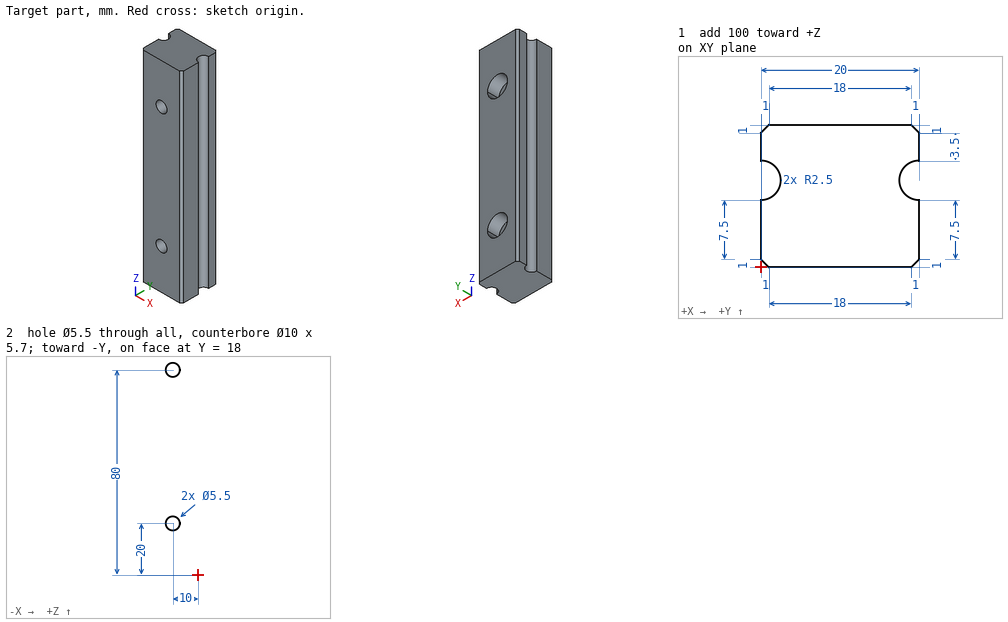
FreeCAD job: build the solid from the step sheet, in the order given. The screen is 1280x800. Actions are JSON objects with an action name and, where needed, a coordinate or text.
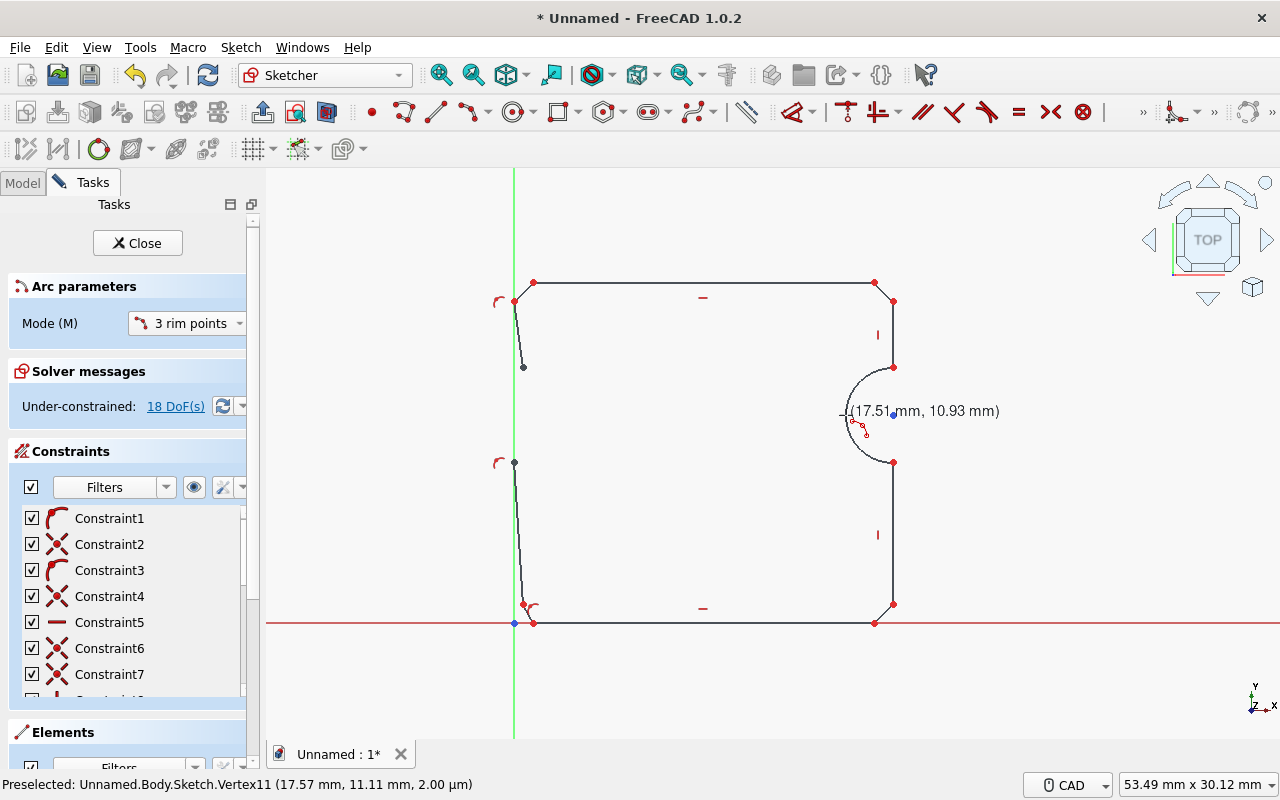
{"action": "left_click", "coordinate": [523, 368]}
{"action": "left_click", "coordinate": [514, 463]}
{"action": "left_click", "coordinate": [561, 415]}
{"action": "key", "text": "Escape"}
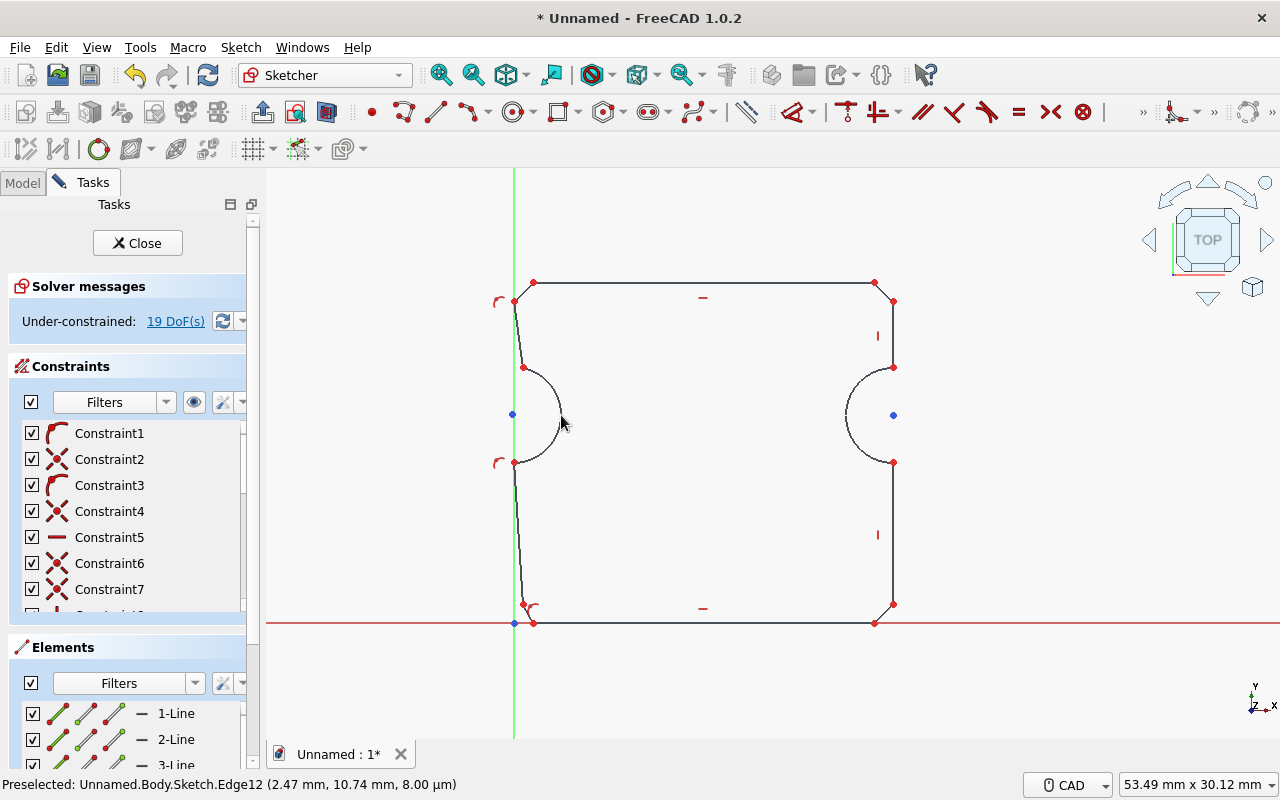
{"action": "left_click", "coordinate": [517, 506]}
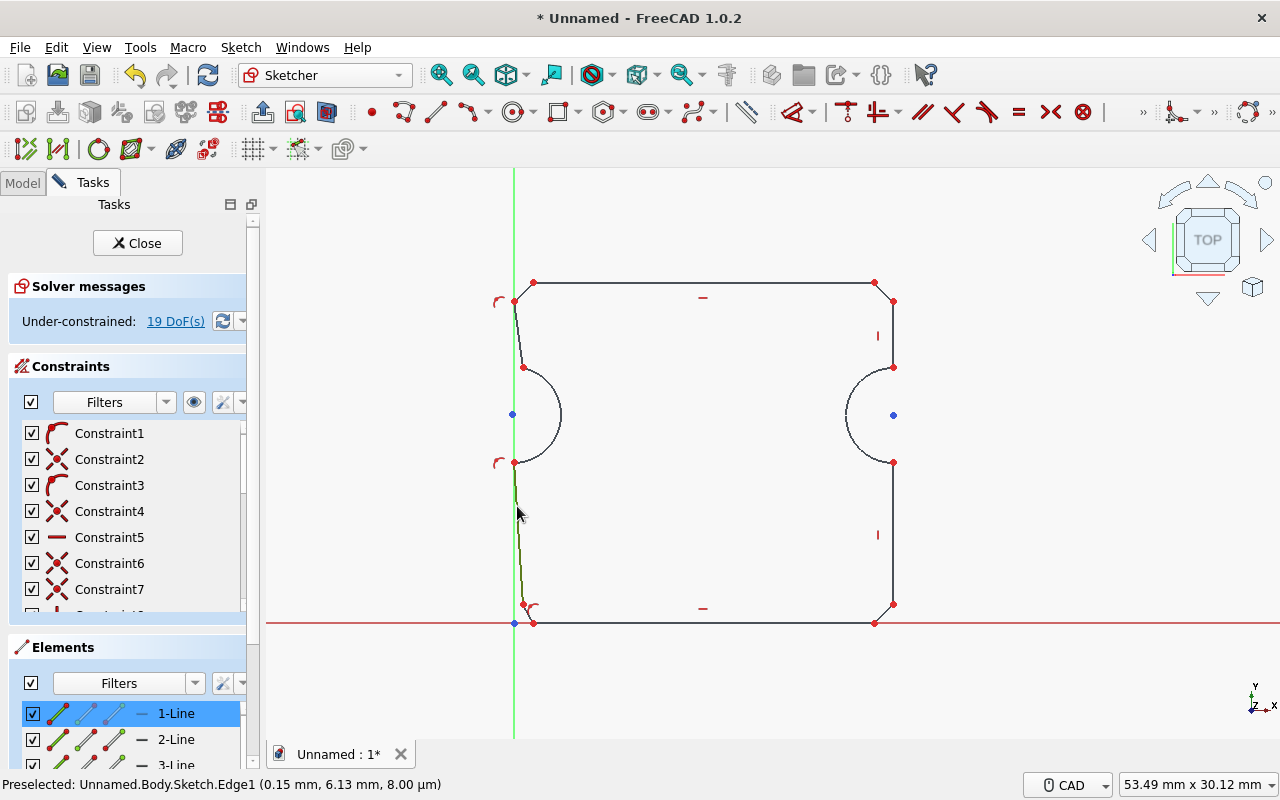
{"action": "key", "text": "v"}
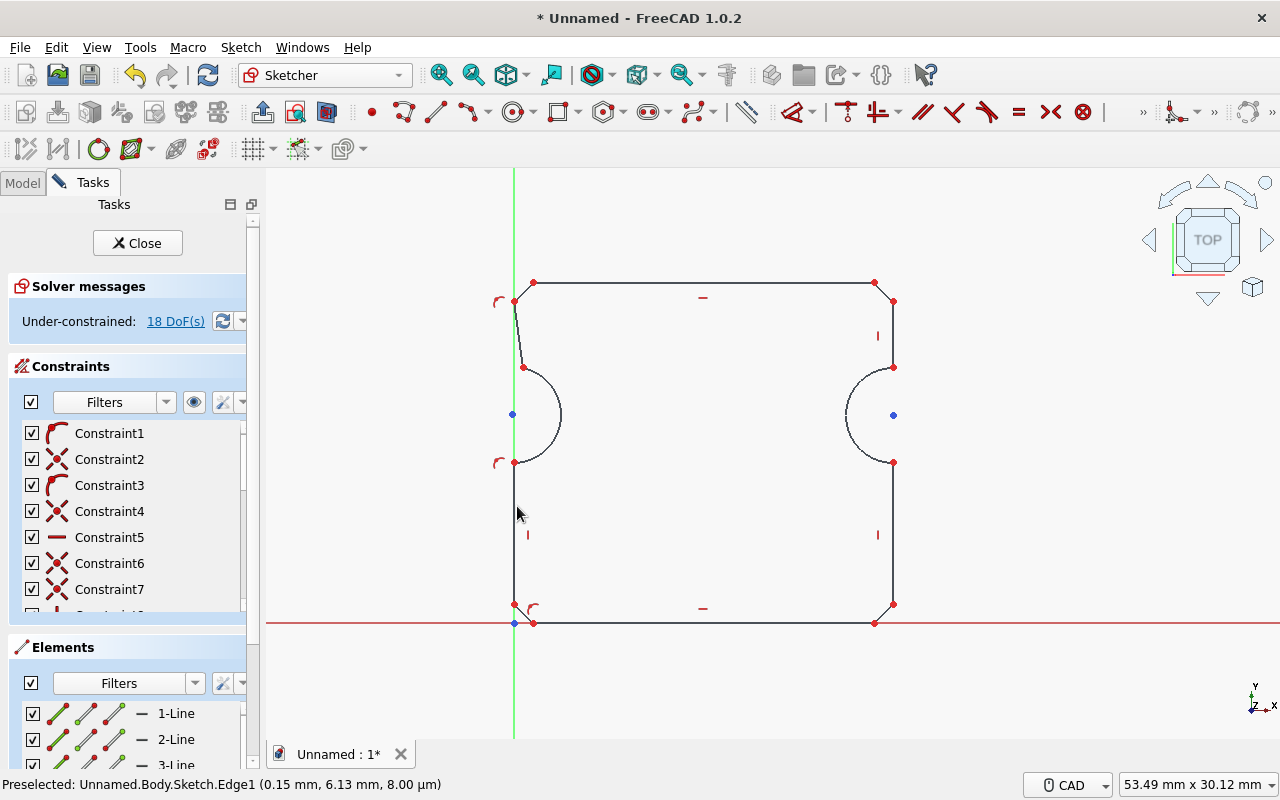
{"action": "left_click", "coordinate": [517, 322]}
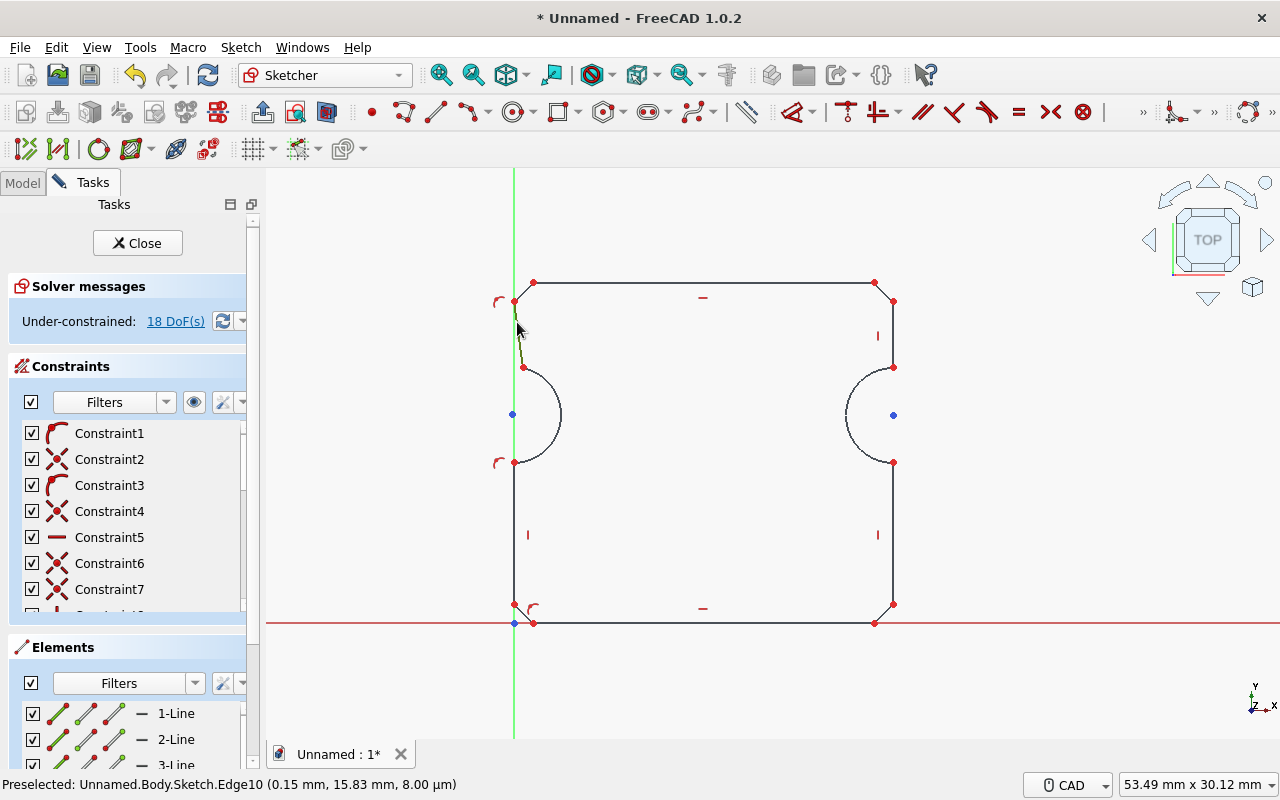
{"action": "key", "text": "v"}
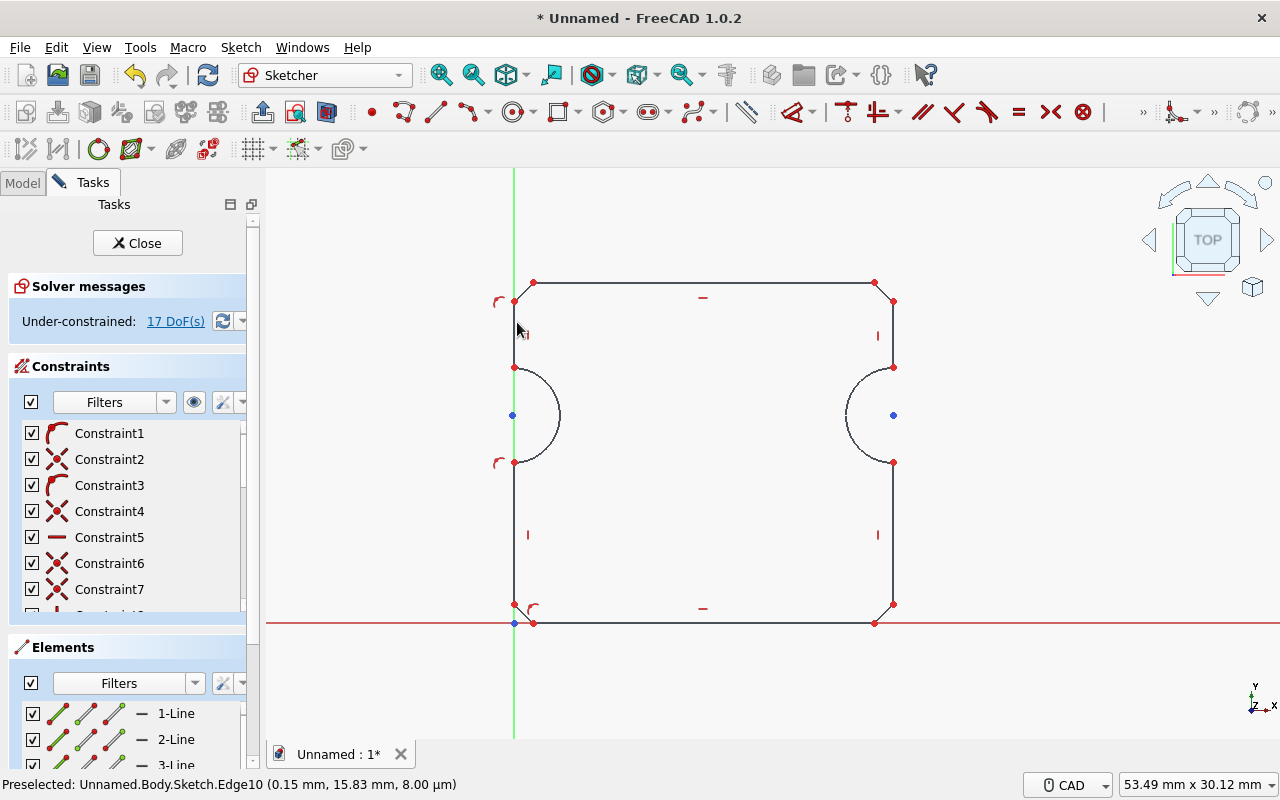
{"action": "left_click", "coordinate": [855, 388]}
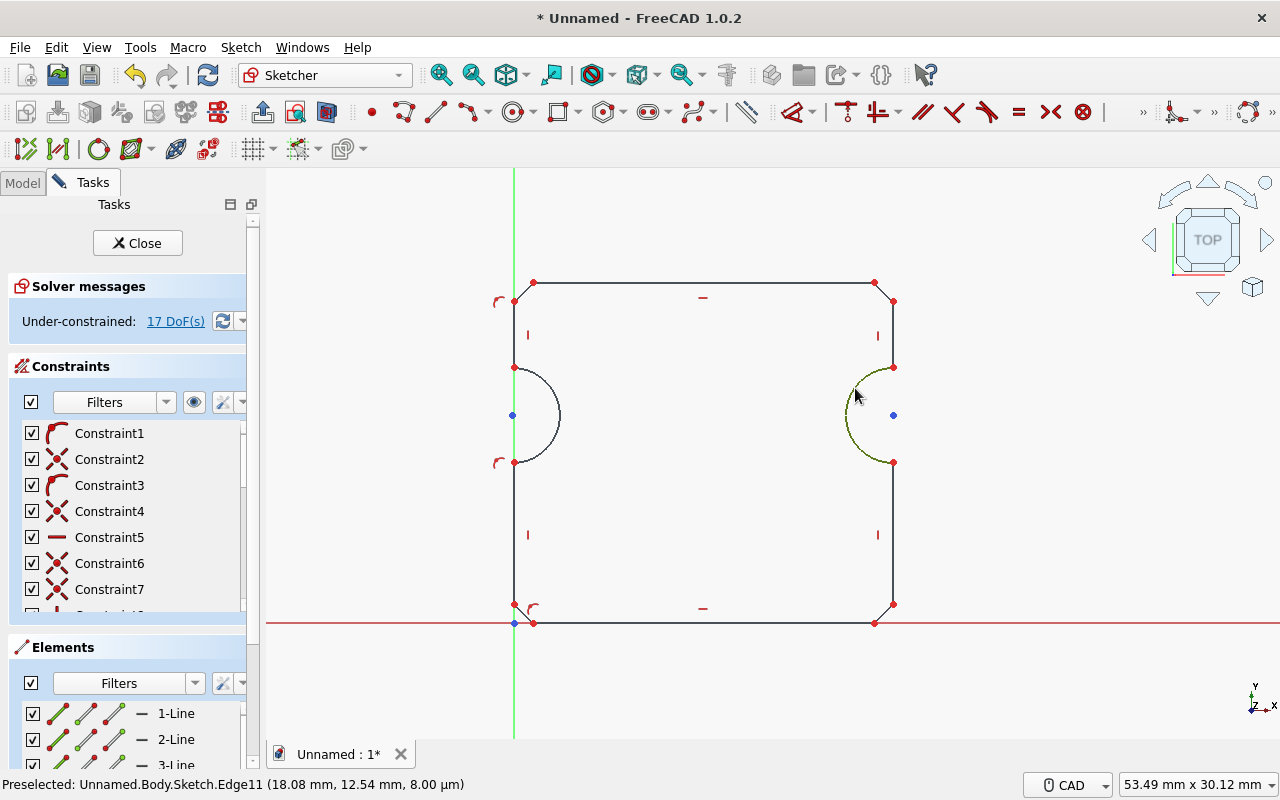
{"action": "left_click", "coordinate": [551, 443]}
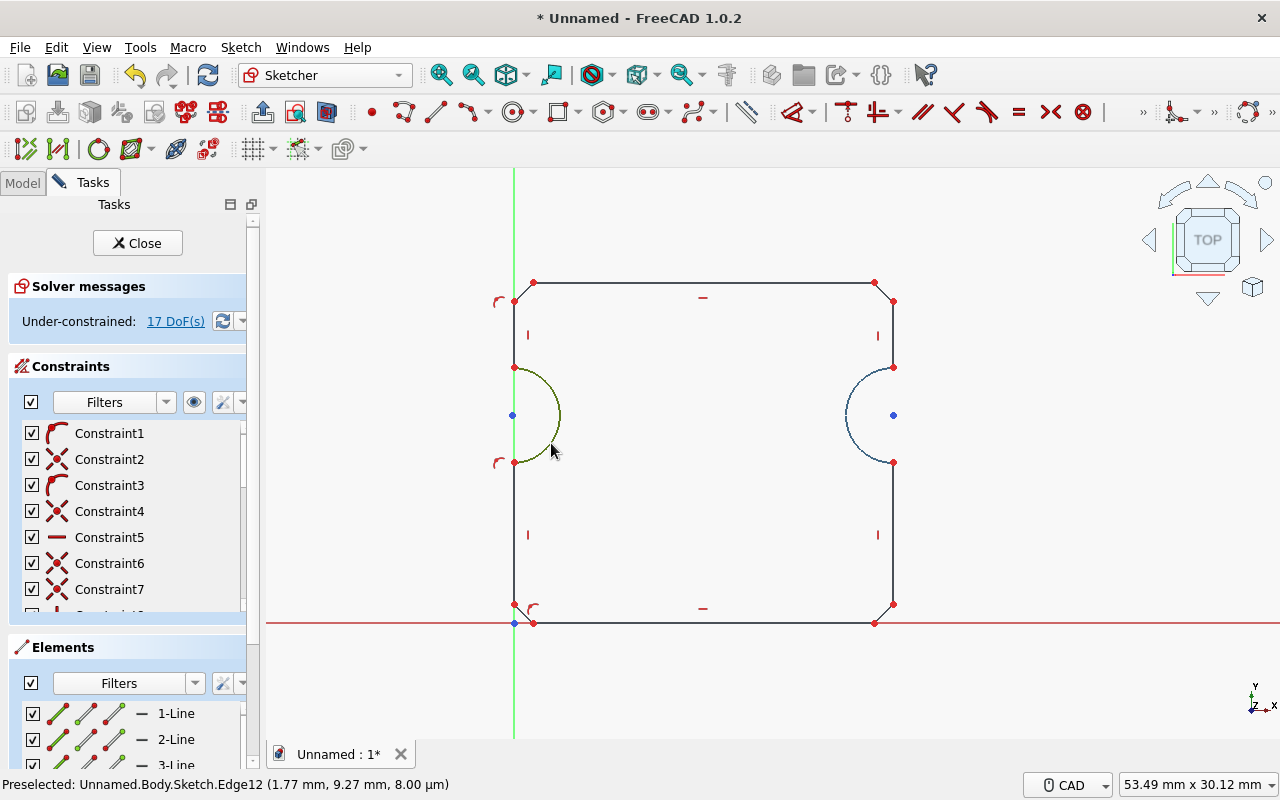
{"action": "left_click", "coordinate": [1020, 112]}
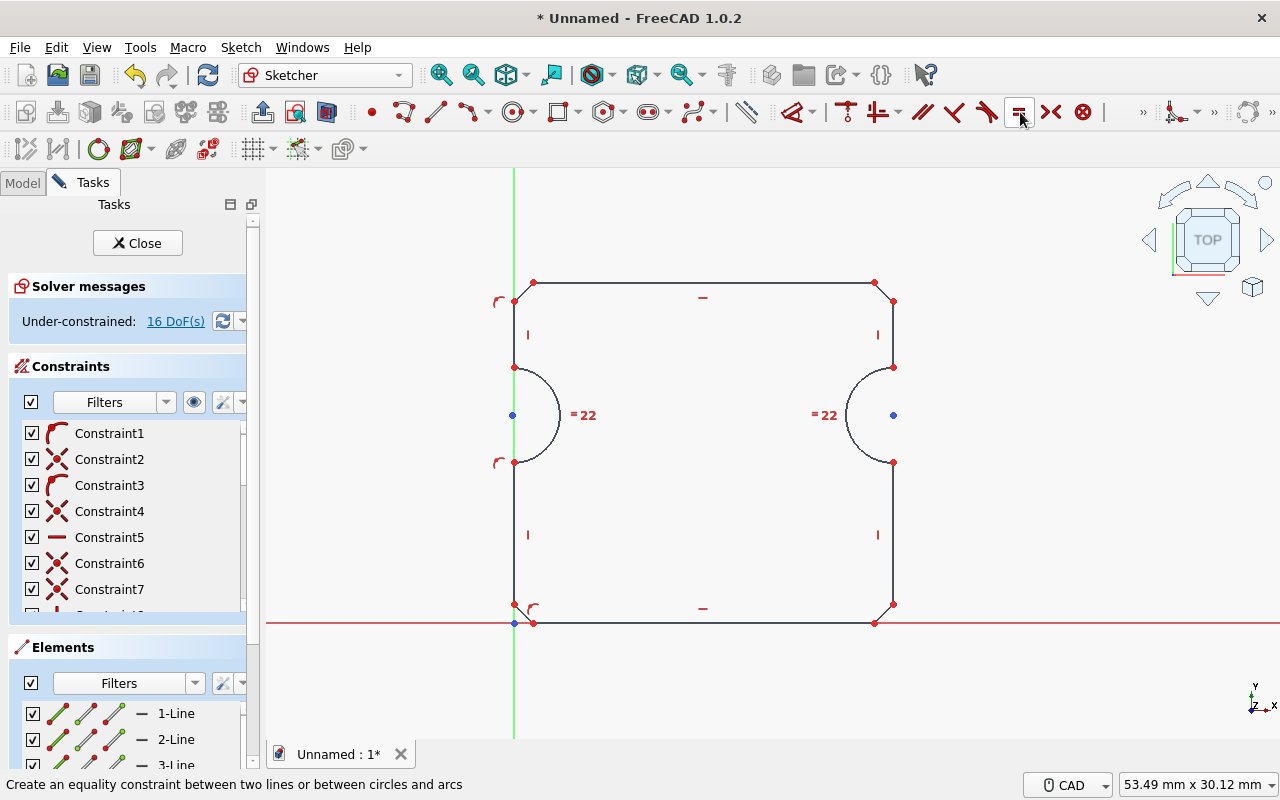
{"action": "left_click", "coordinate": [512, 415]}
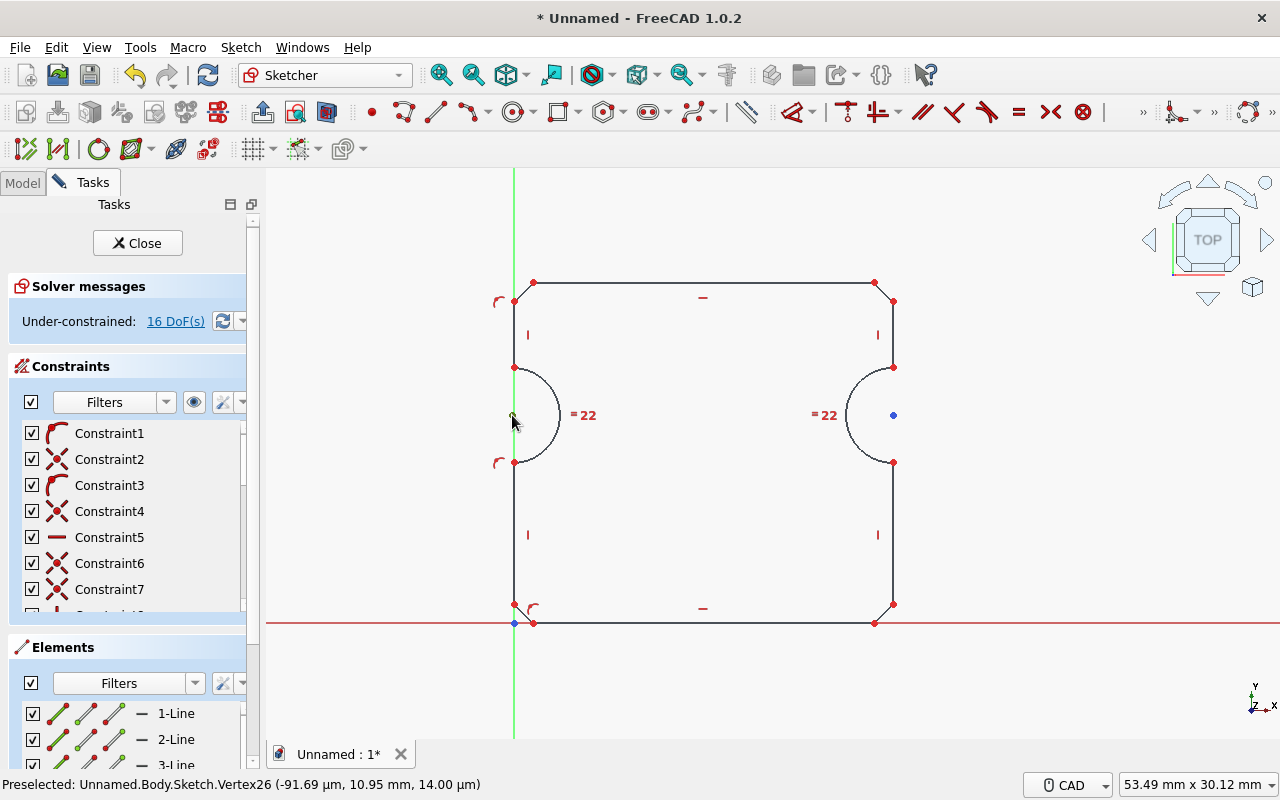
{"action": "left_click", "coordinate": [514, 674]}